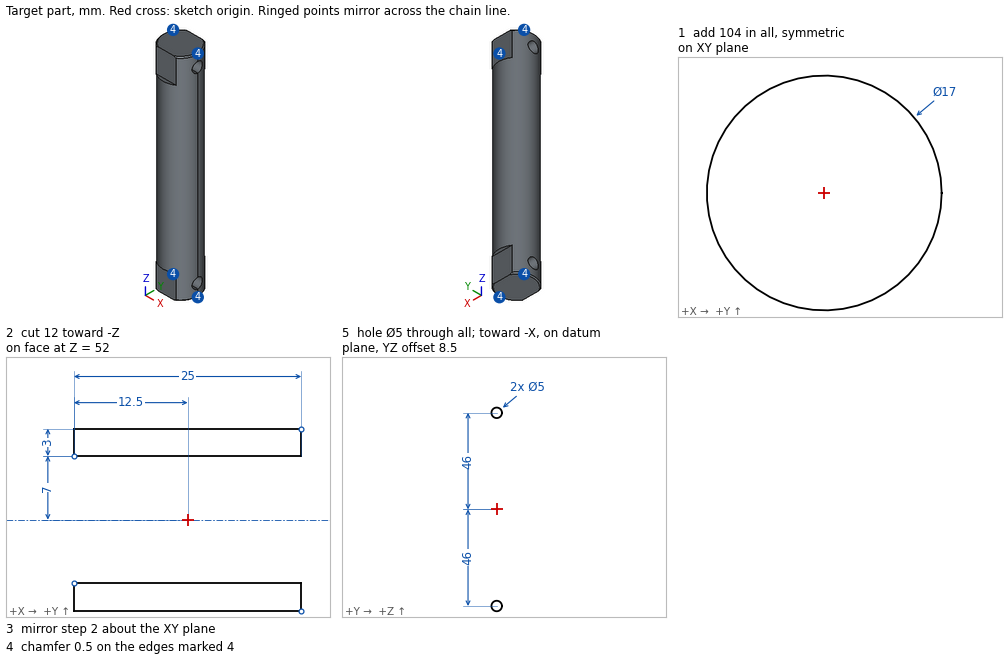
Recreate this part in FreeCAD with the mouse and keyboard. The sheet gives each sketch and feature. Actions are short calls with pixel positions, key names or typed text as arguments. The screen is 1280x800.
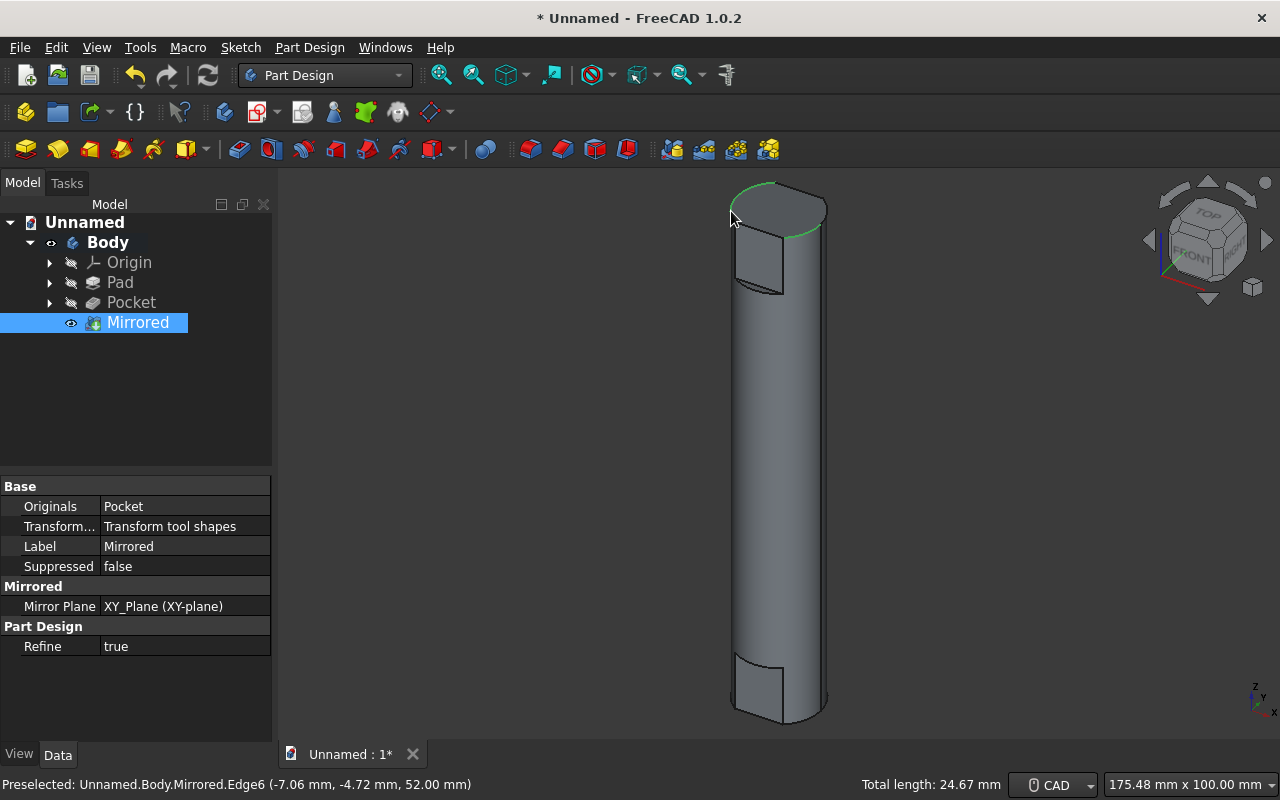
key(0)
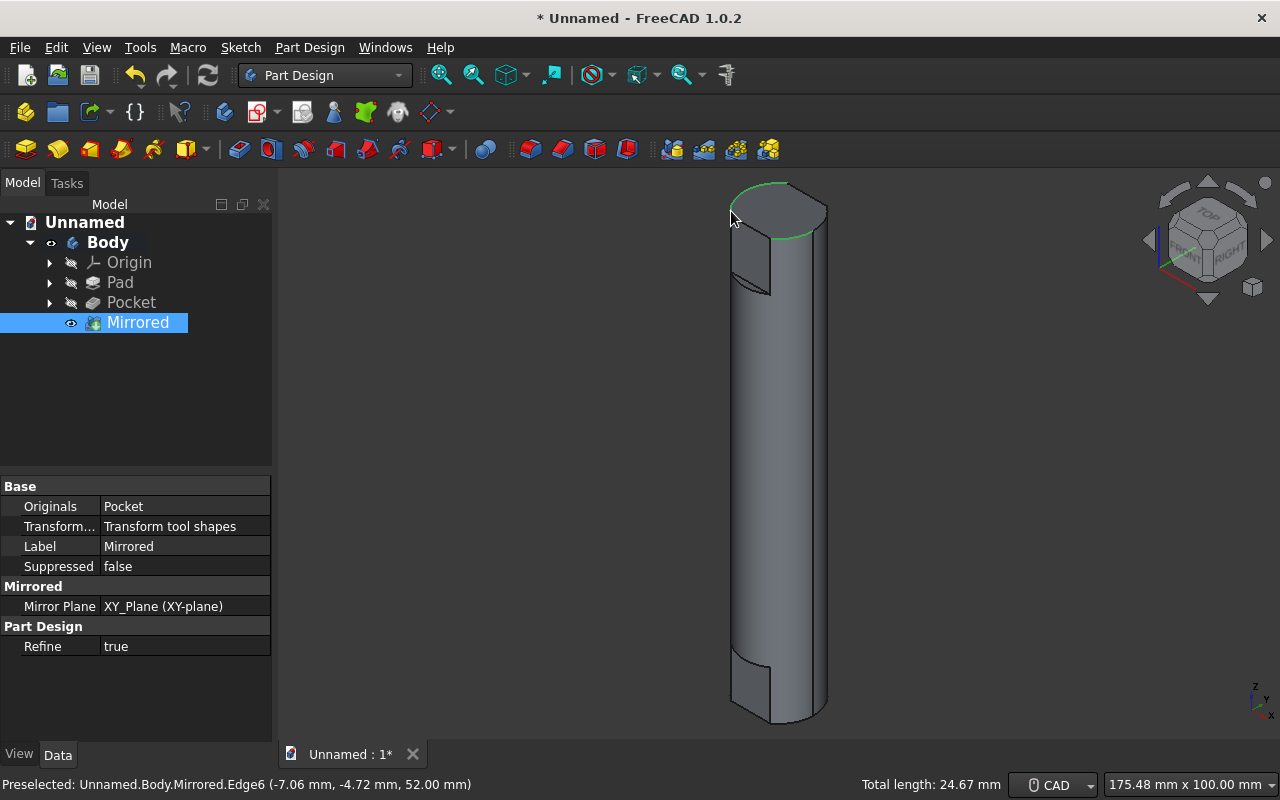
click(822, 708, ctrl)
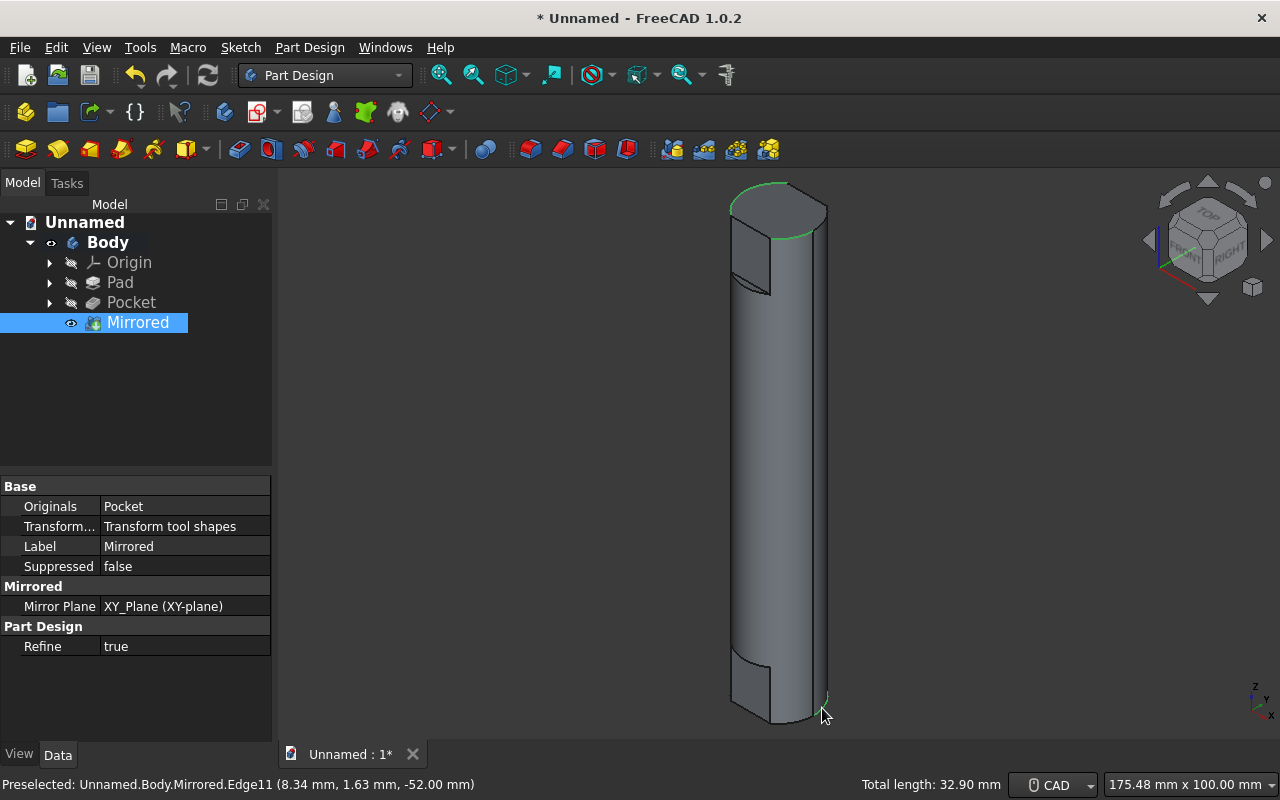
key(2)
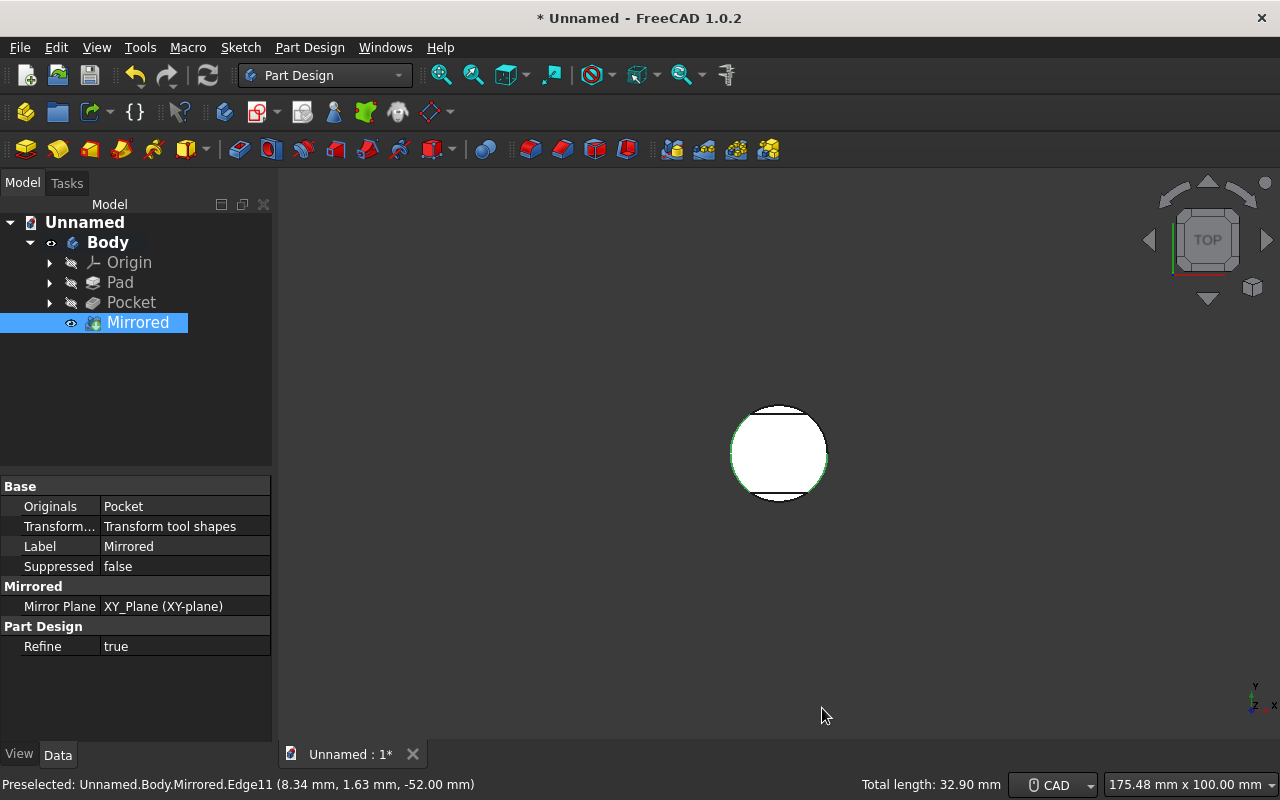
click(442, 76)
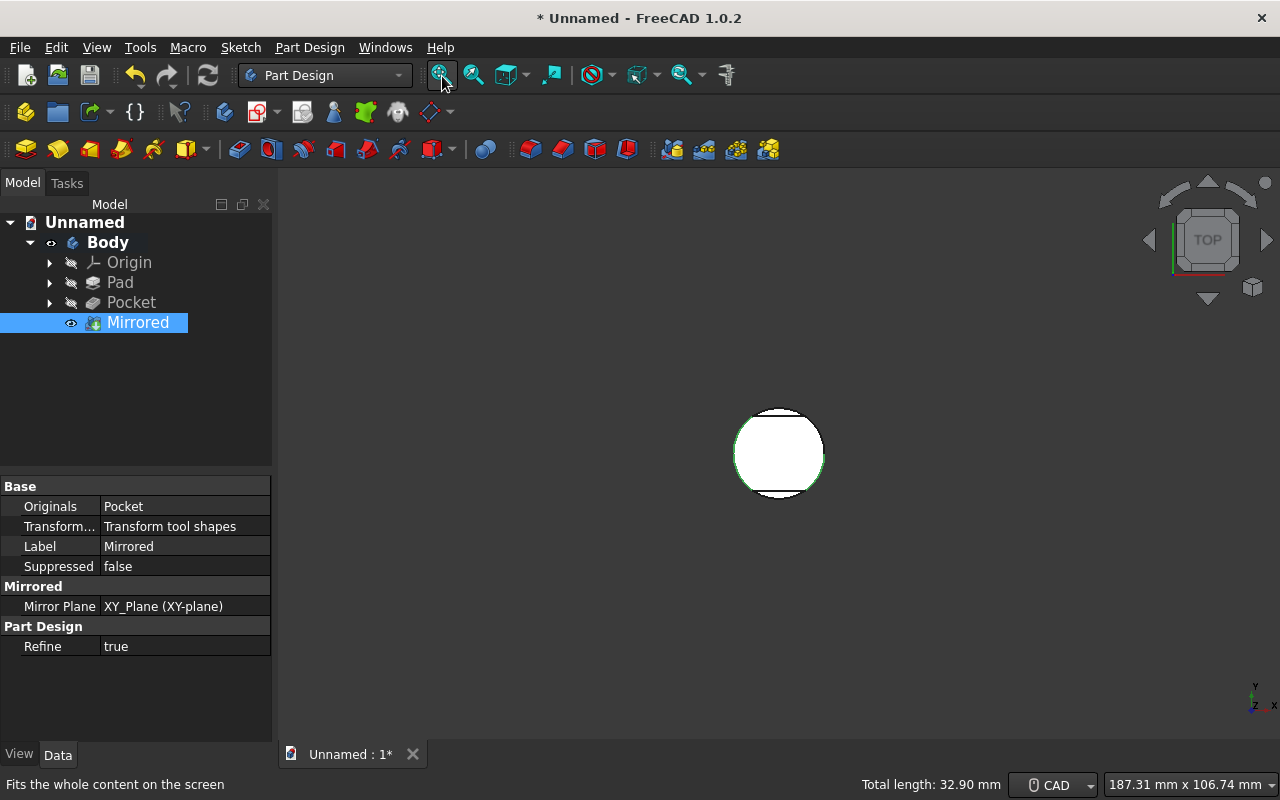
key(1)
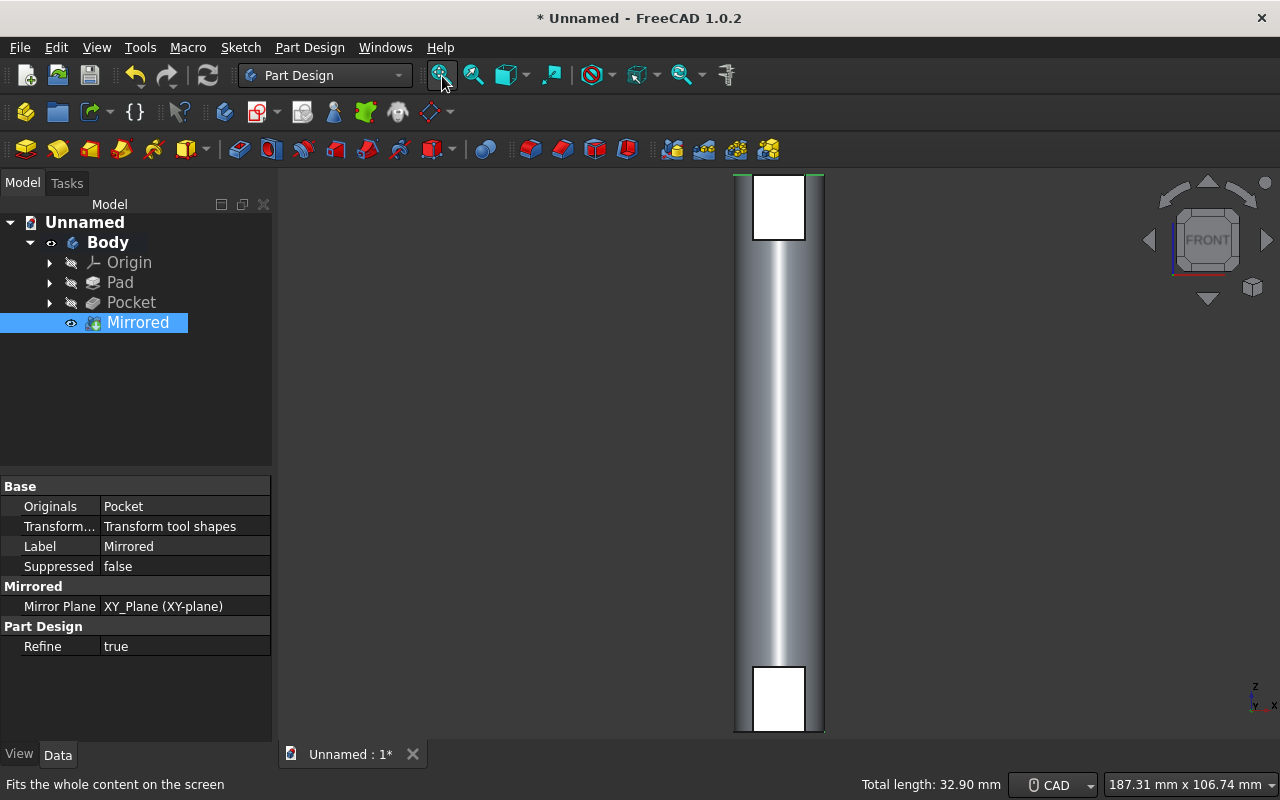
key(3)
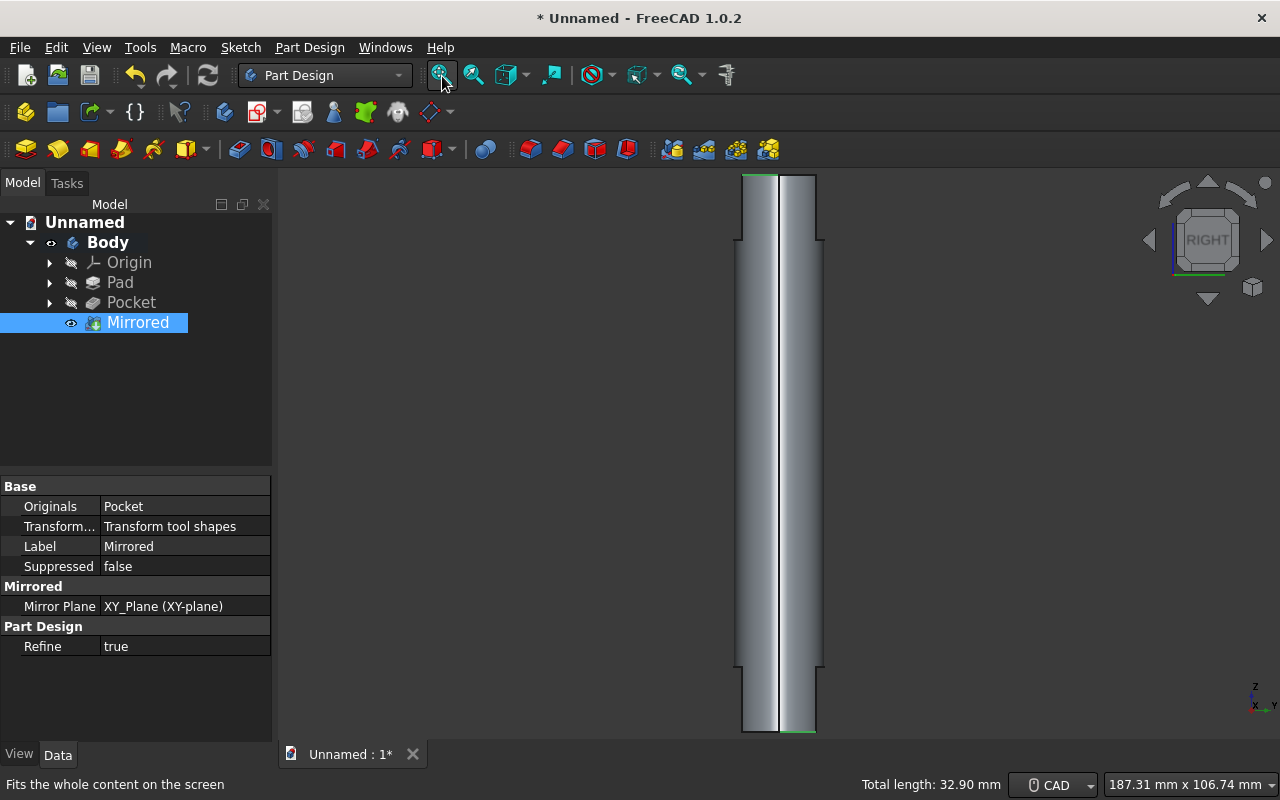
key(5)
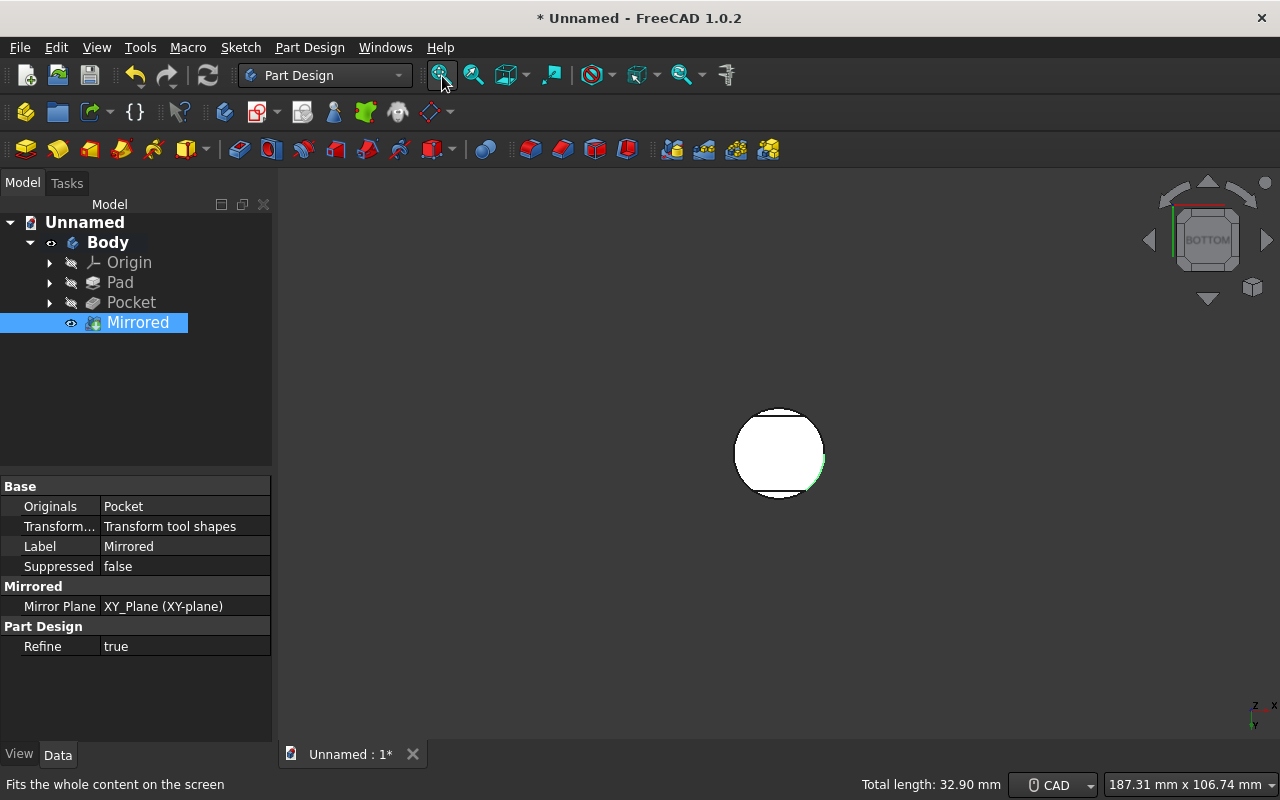
click(442, 76)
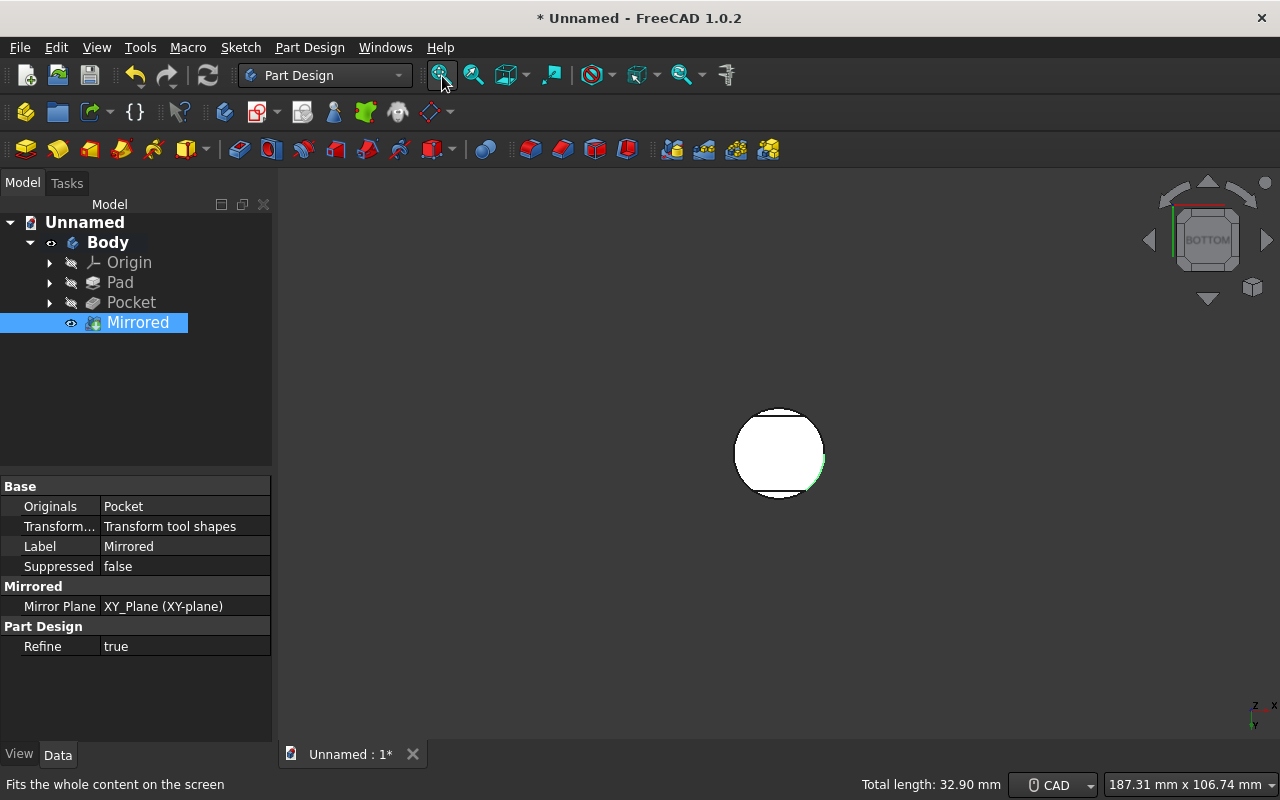
click(734, 452, ctrl)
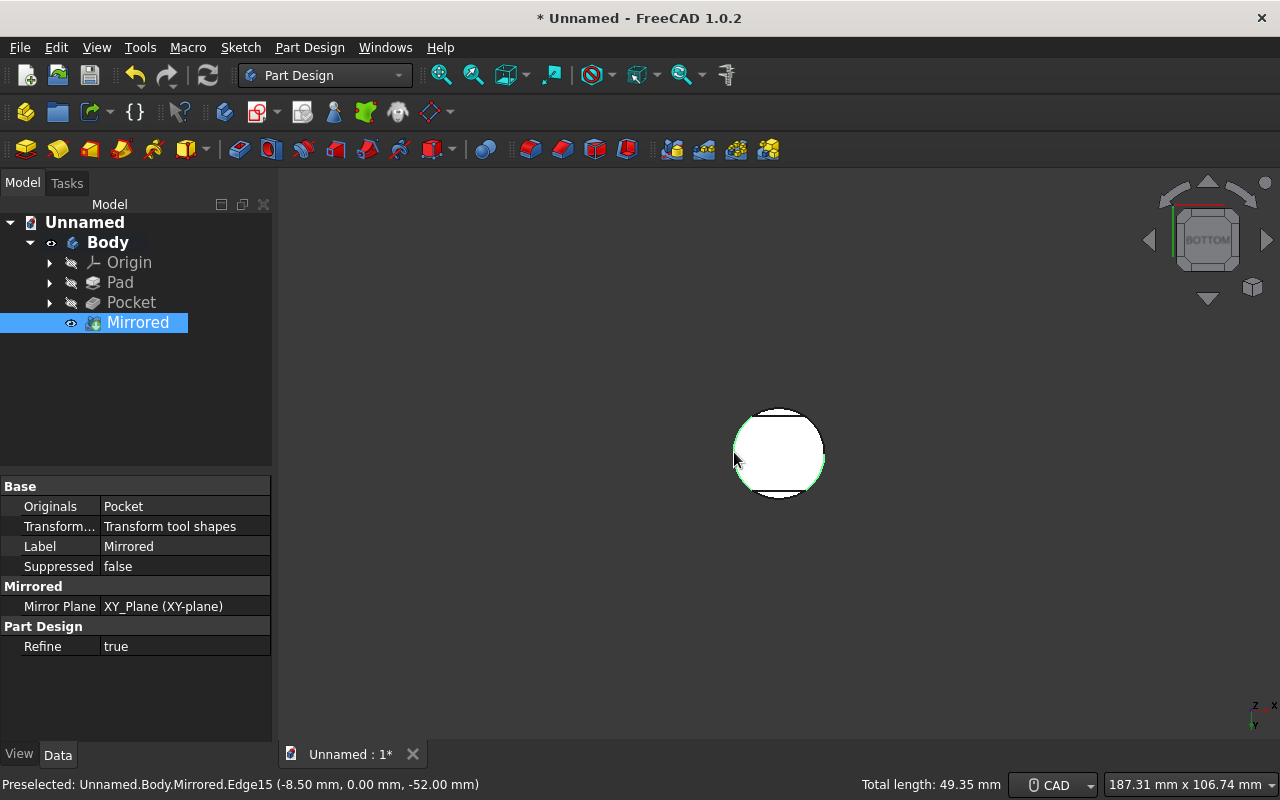
click(564, 150)